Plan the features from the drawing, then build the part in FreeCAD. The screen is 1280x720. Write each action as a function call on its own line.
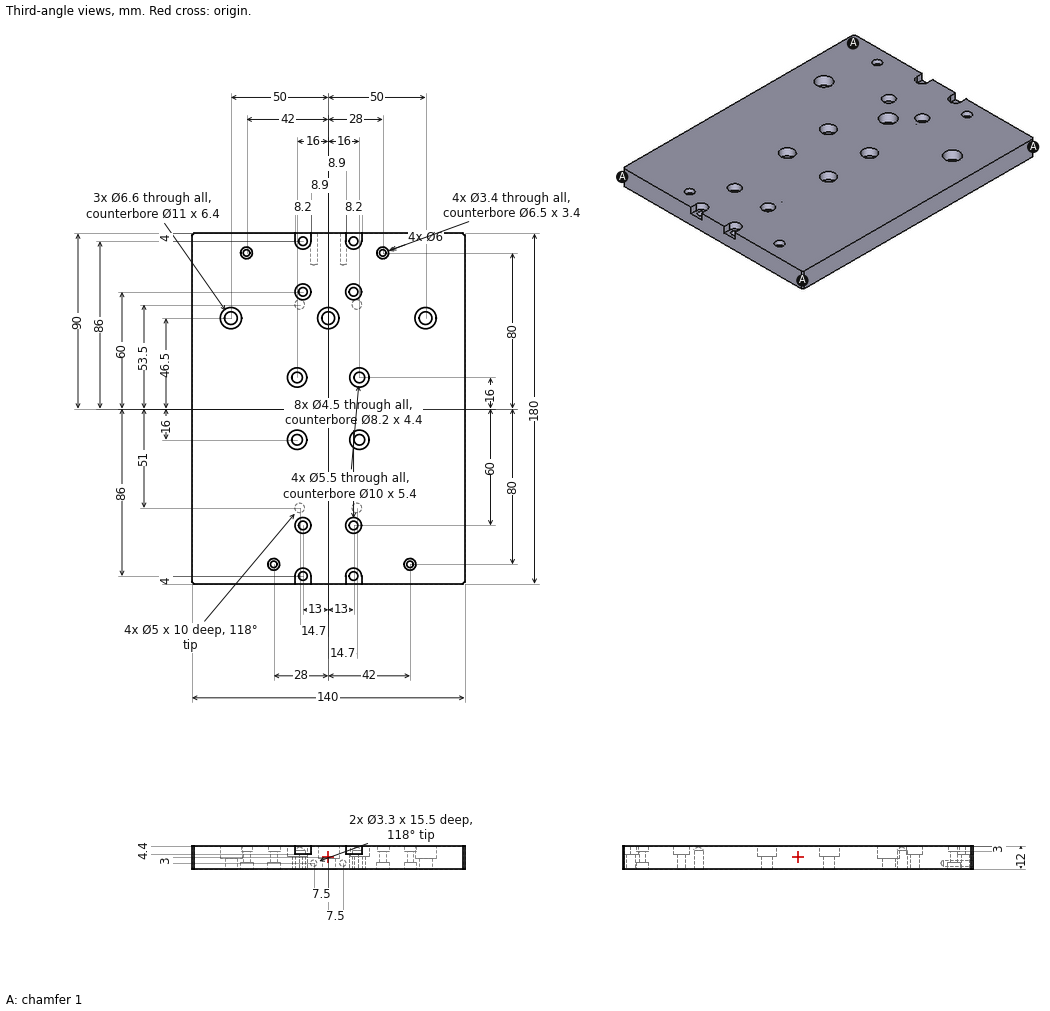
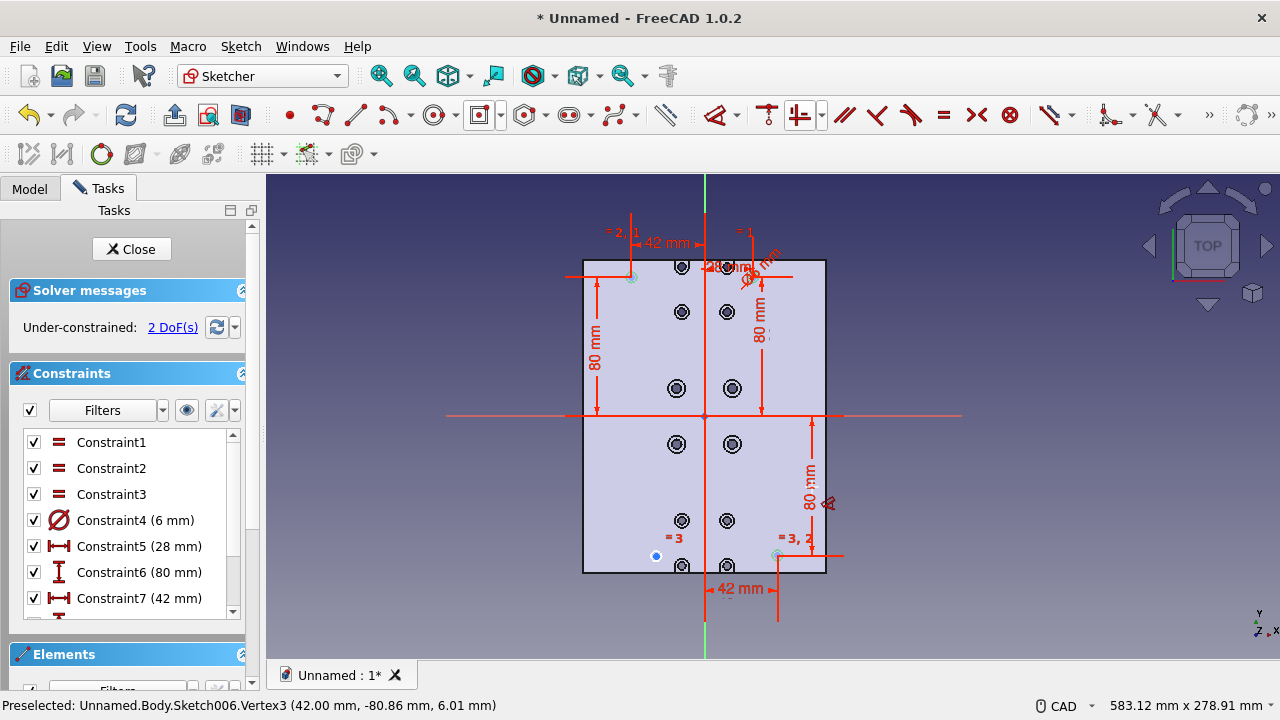
click(656, 556)
click(669, 590)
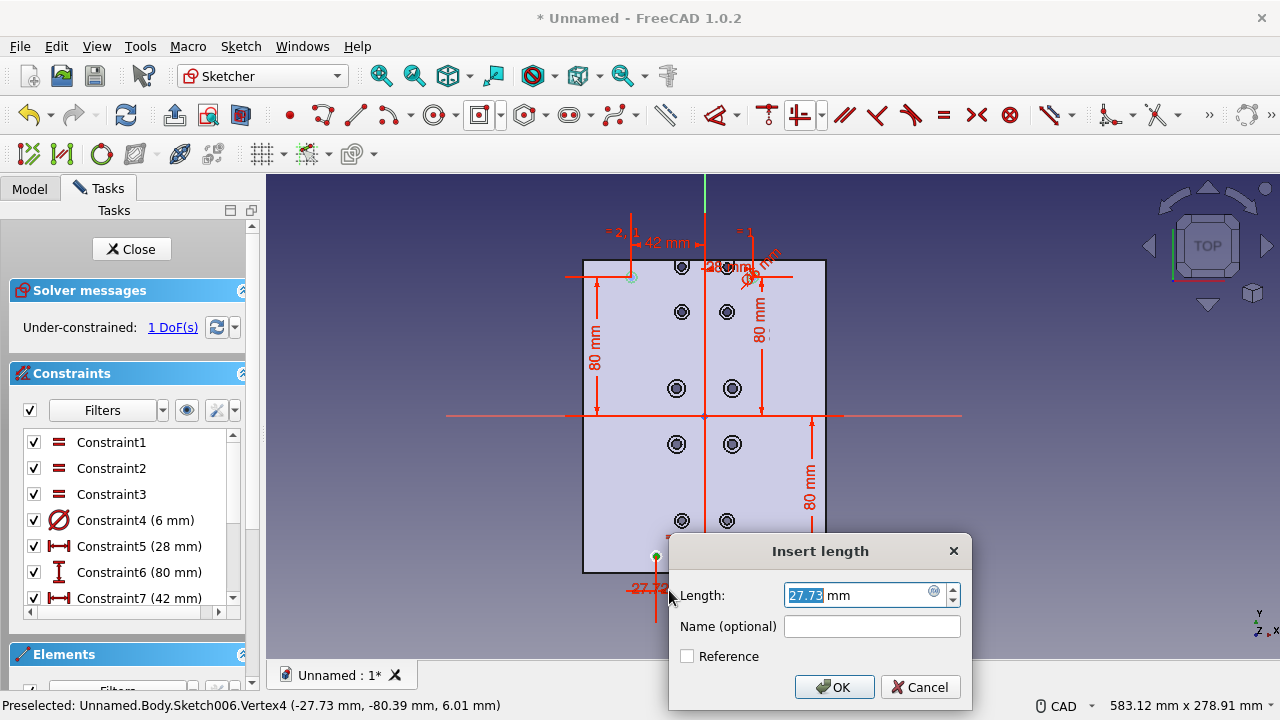
text(28)
key(Return)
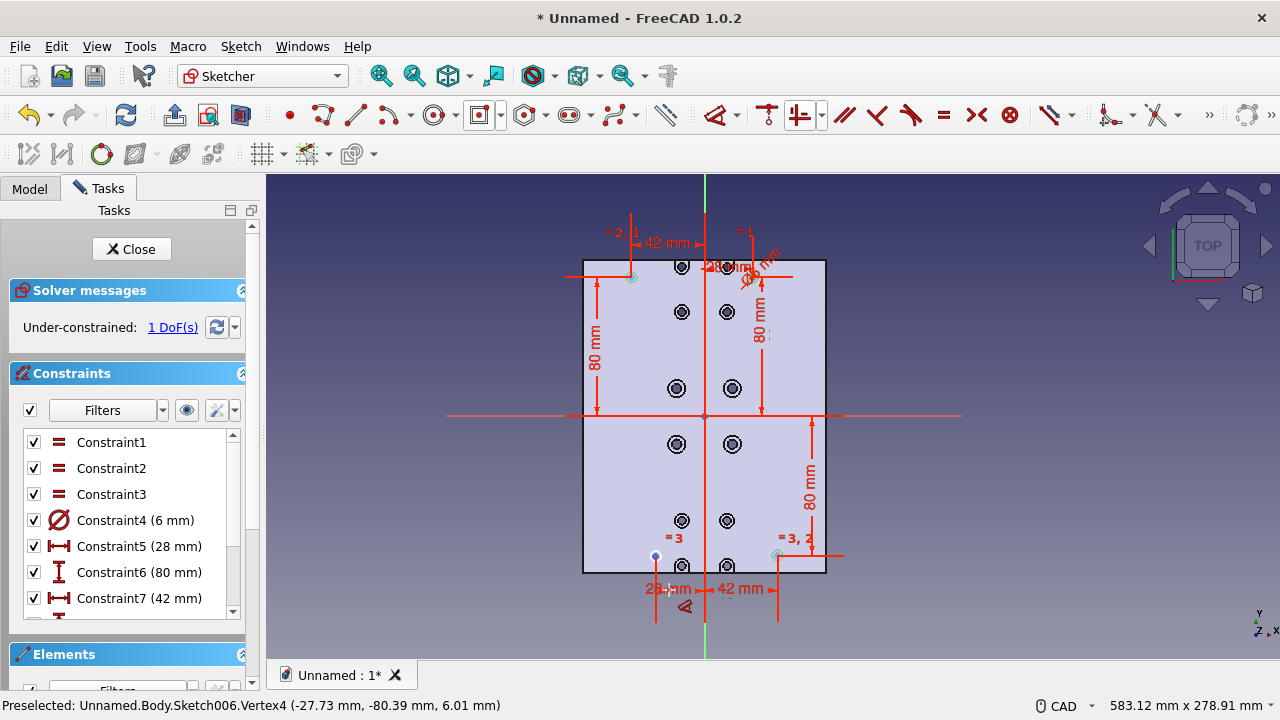
click(656, 556)
click(622, 486)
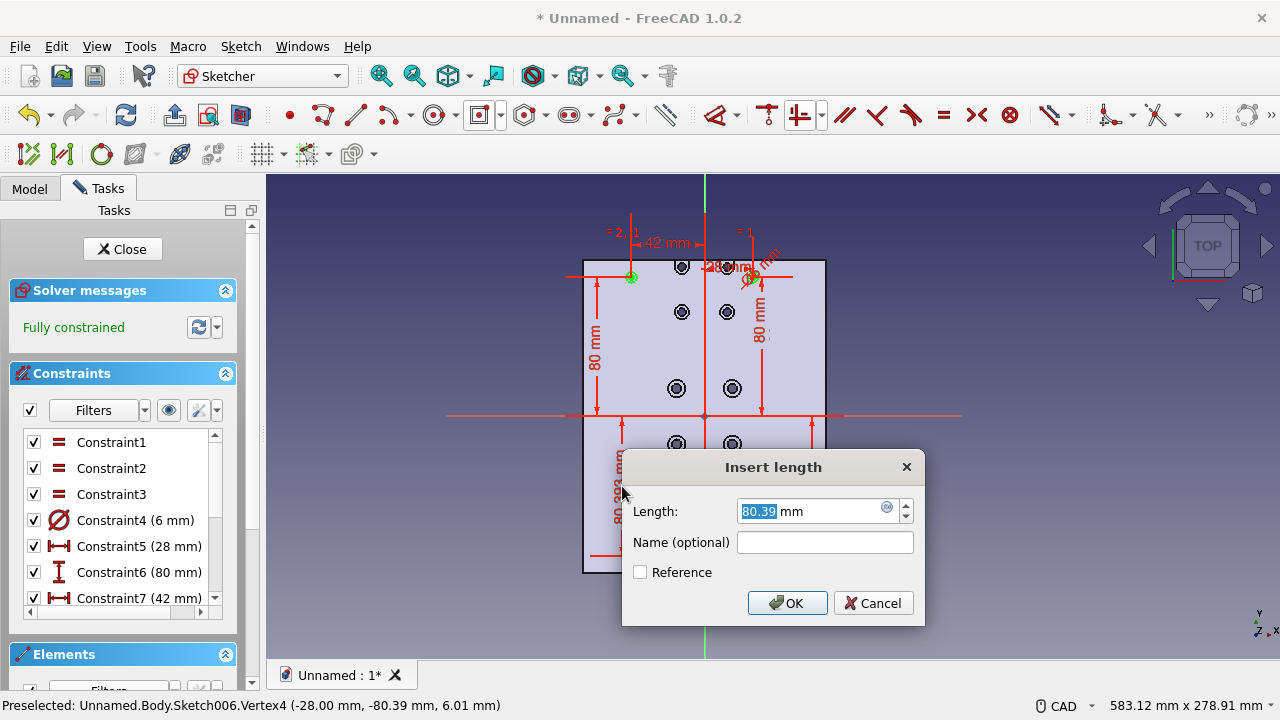
text(80)
key(Return)
key(Escape)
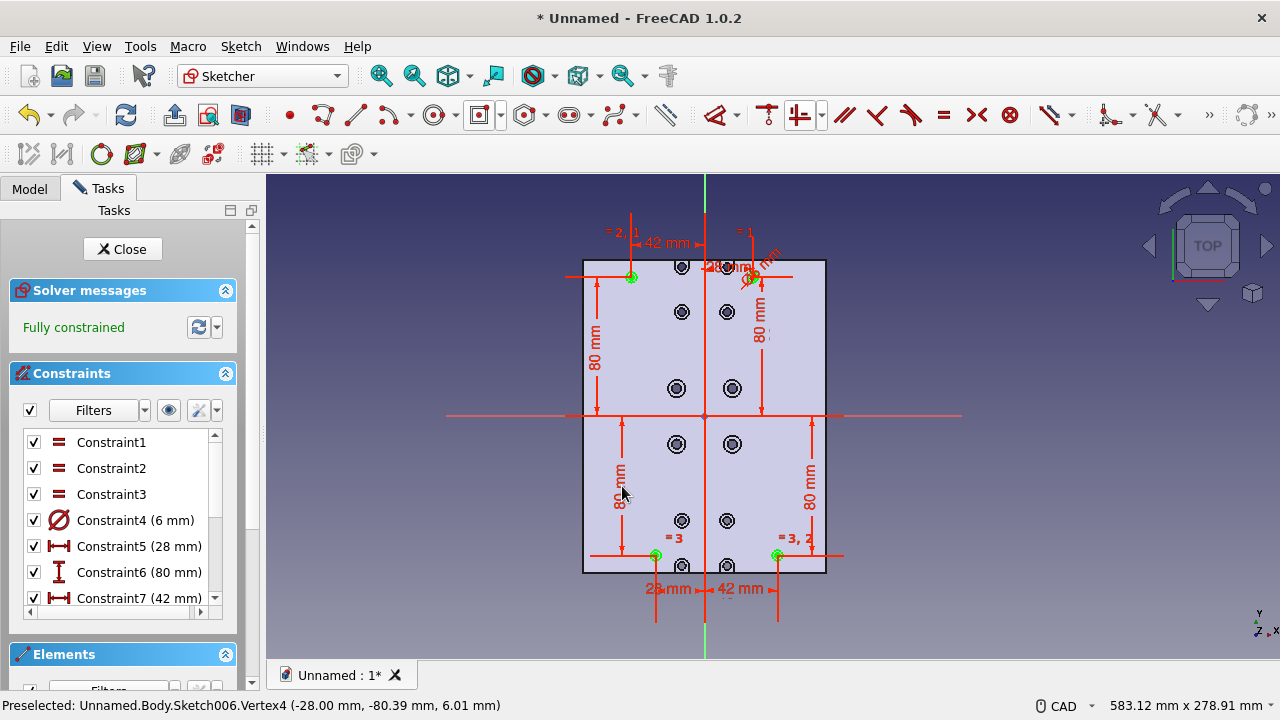
click(123, 249)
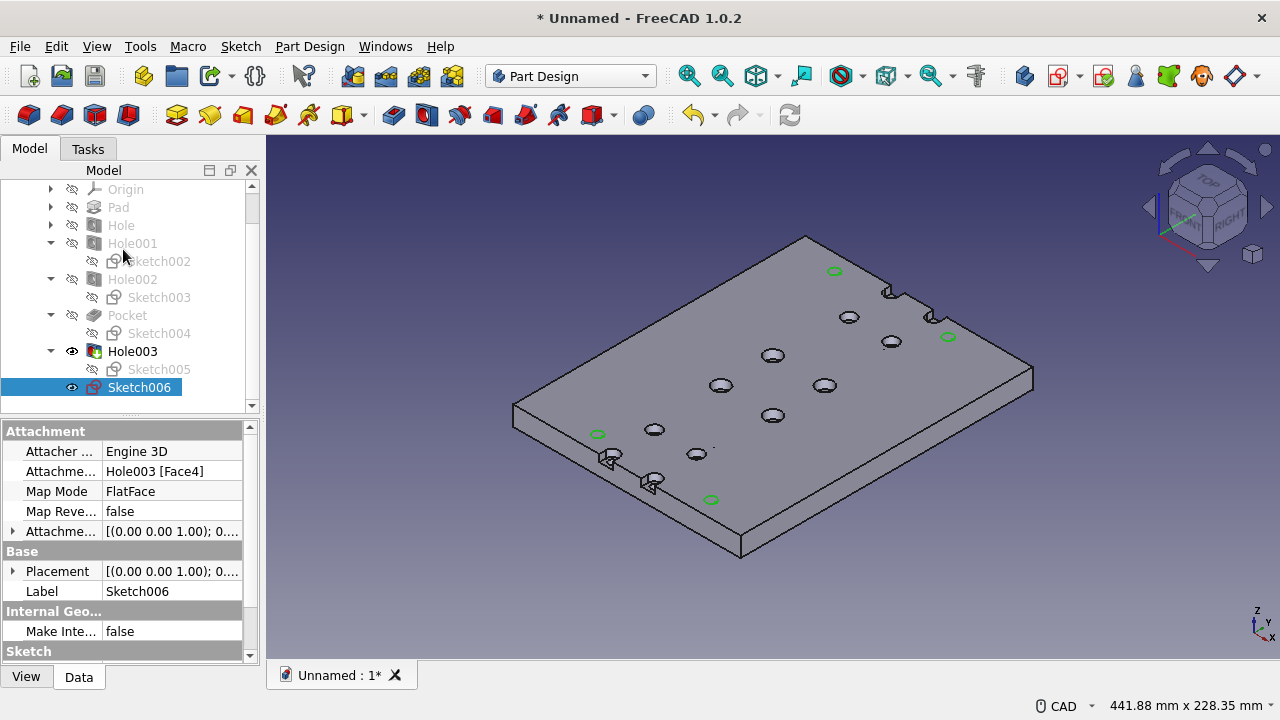
click(394, 116)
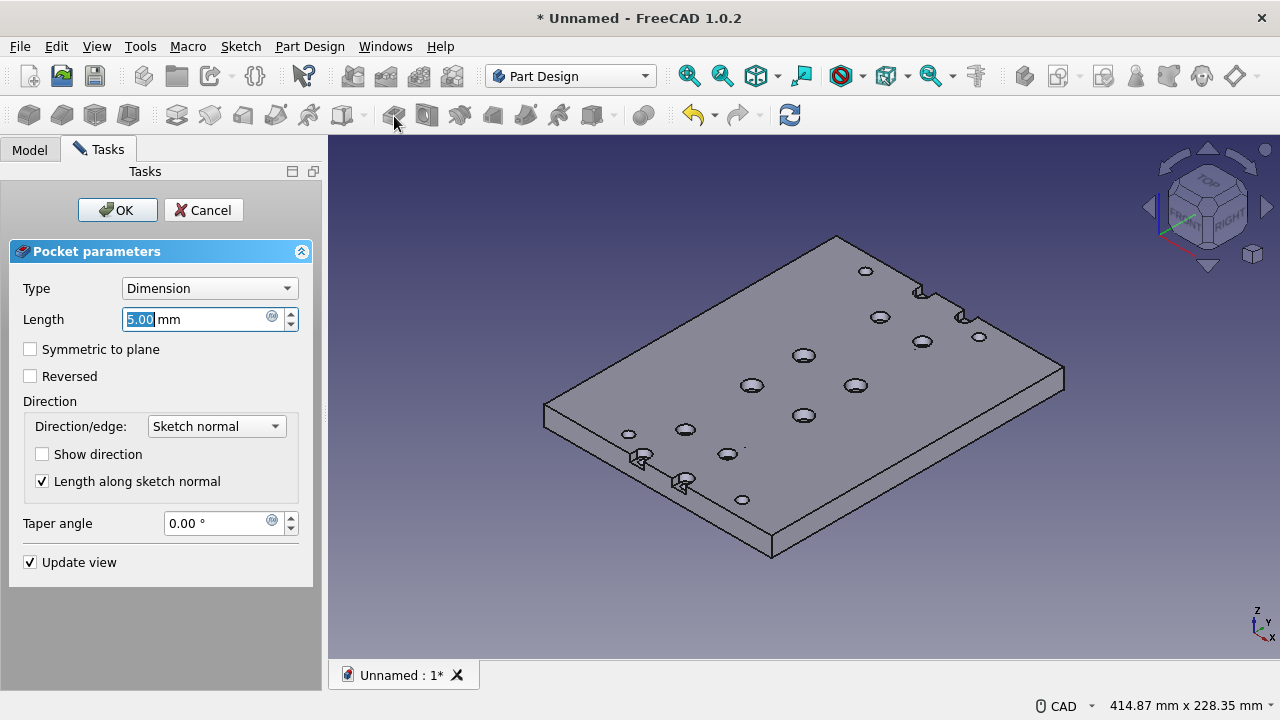
text(3)
key(Tab)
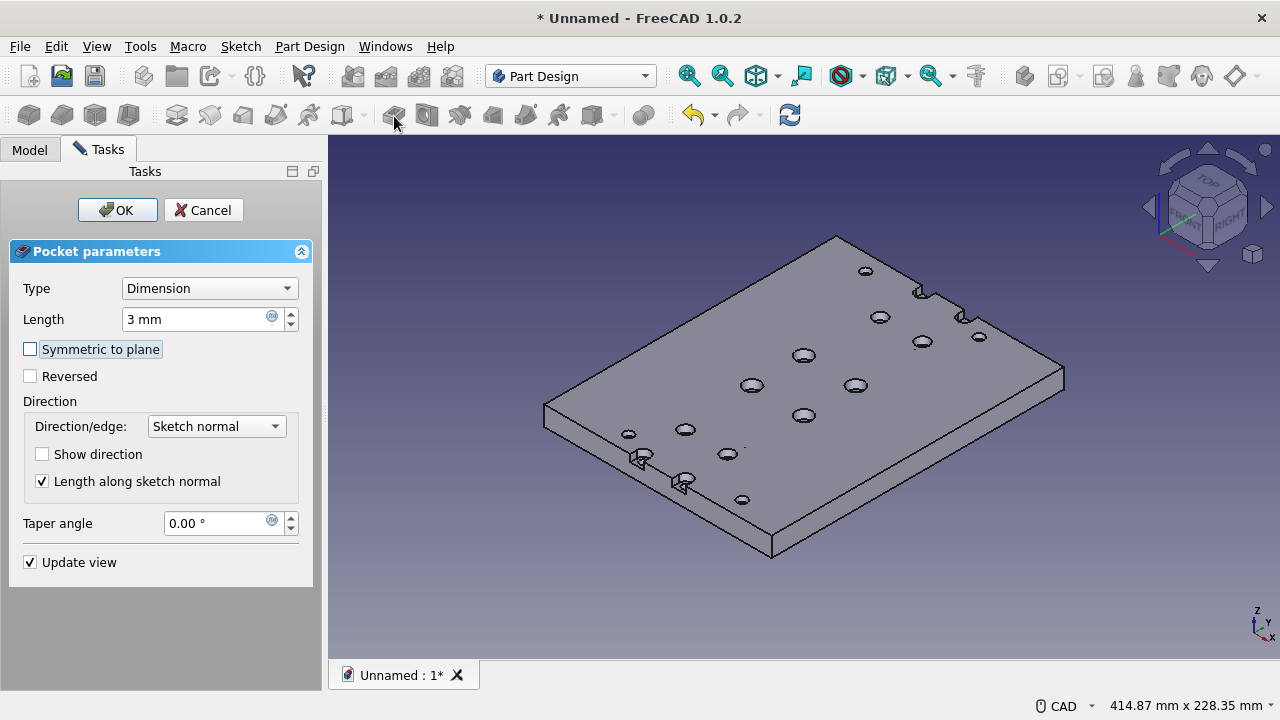
click(118, 210)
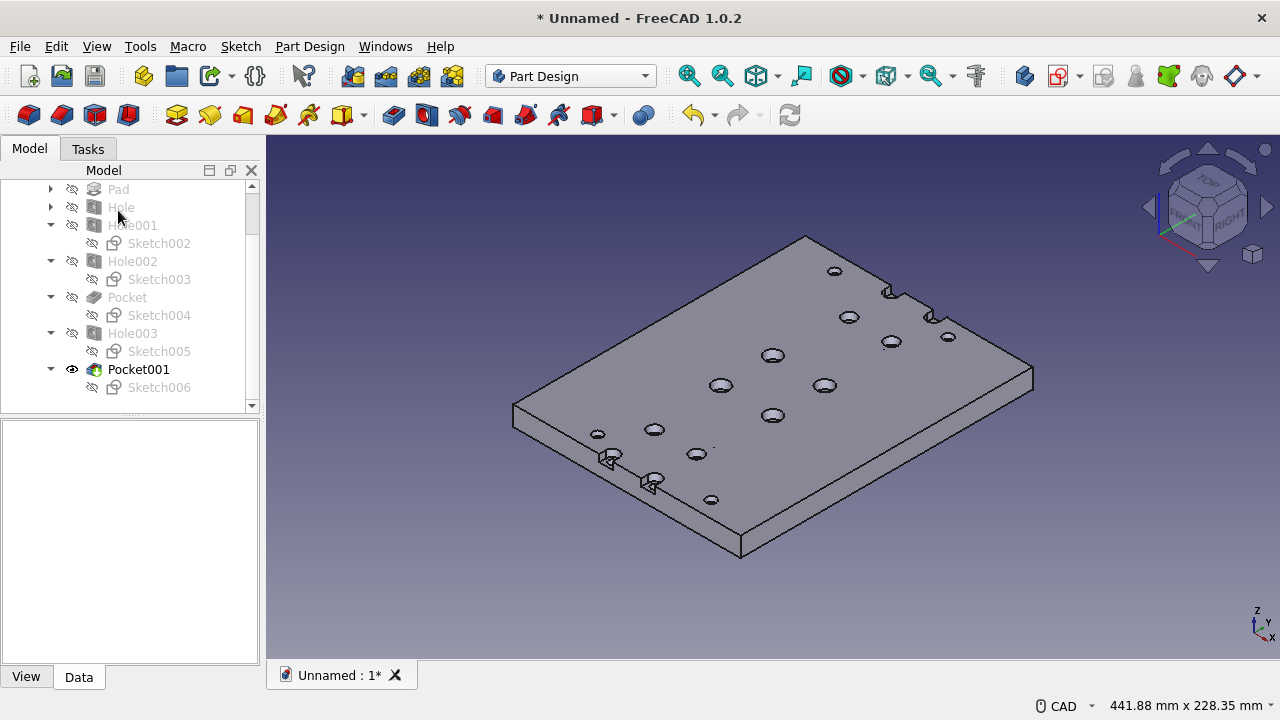
key(5)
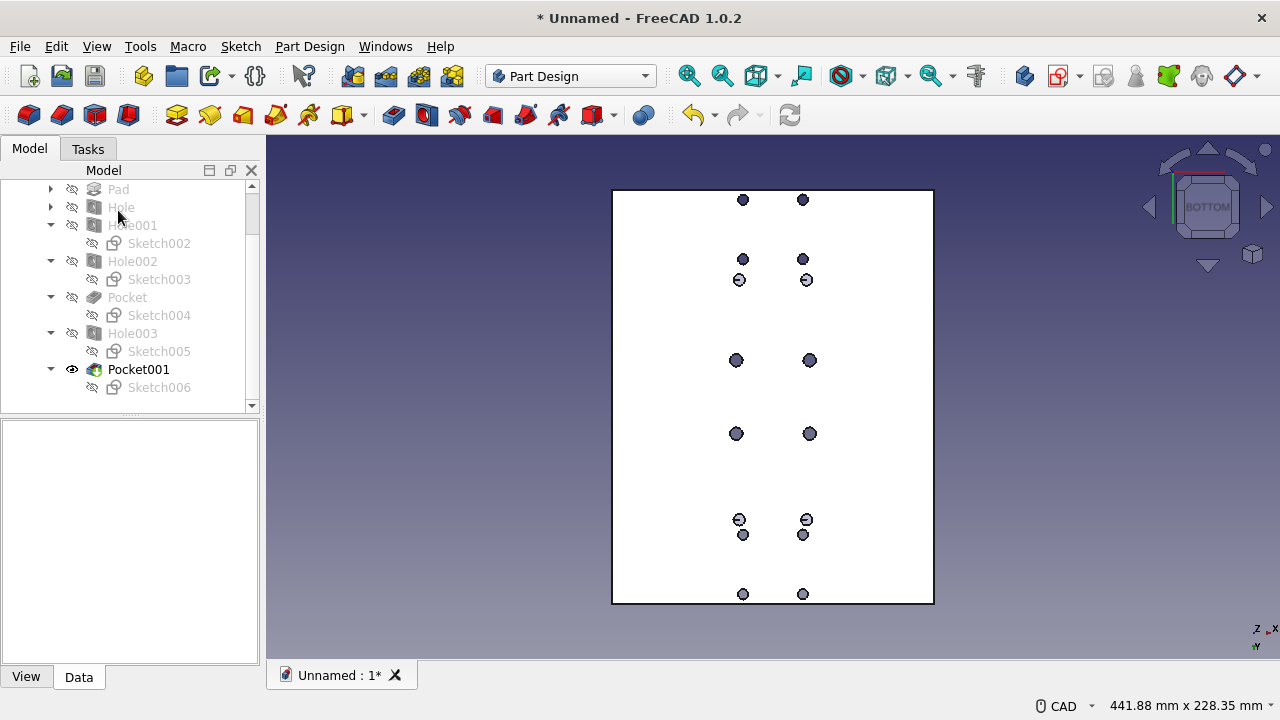
click(865, 396)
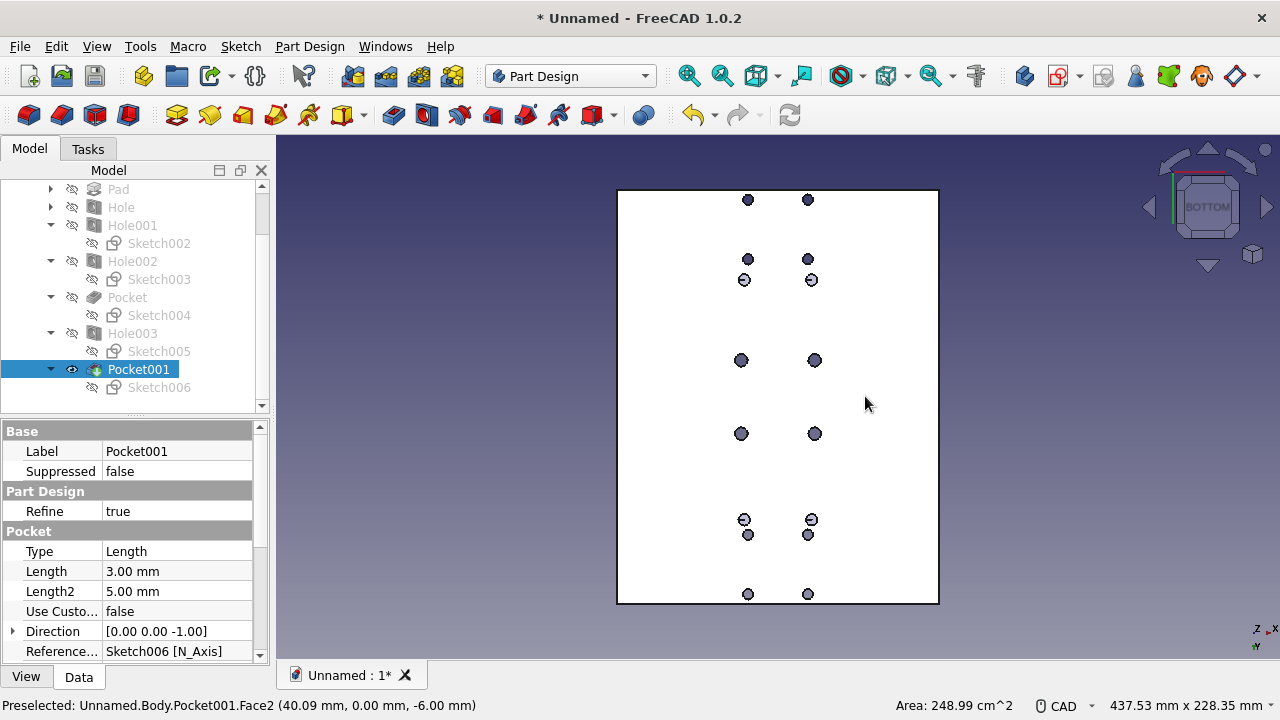
click(1058, 76)